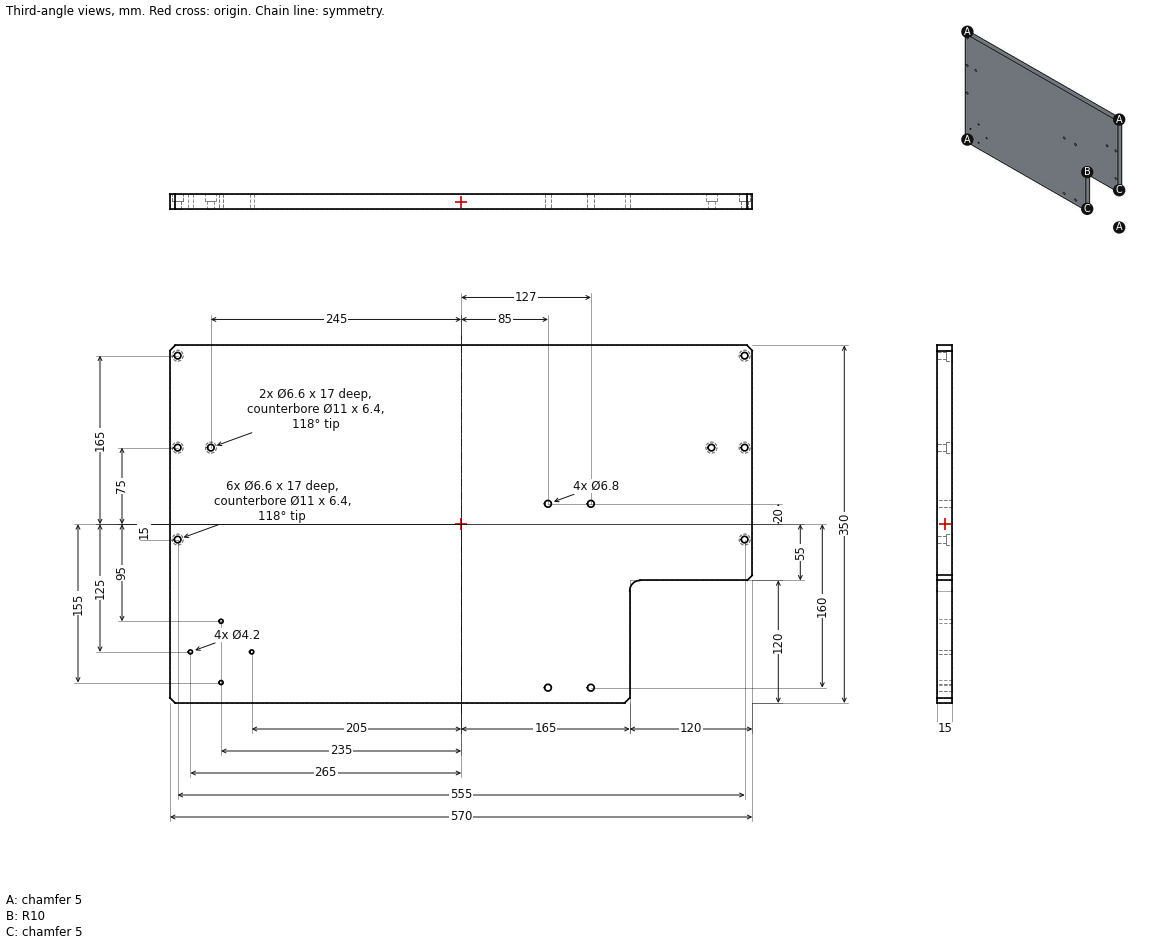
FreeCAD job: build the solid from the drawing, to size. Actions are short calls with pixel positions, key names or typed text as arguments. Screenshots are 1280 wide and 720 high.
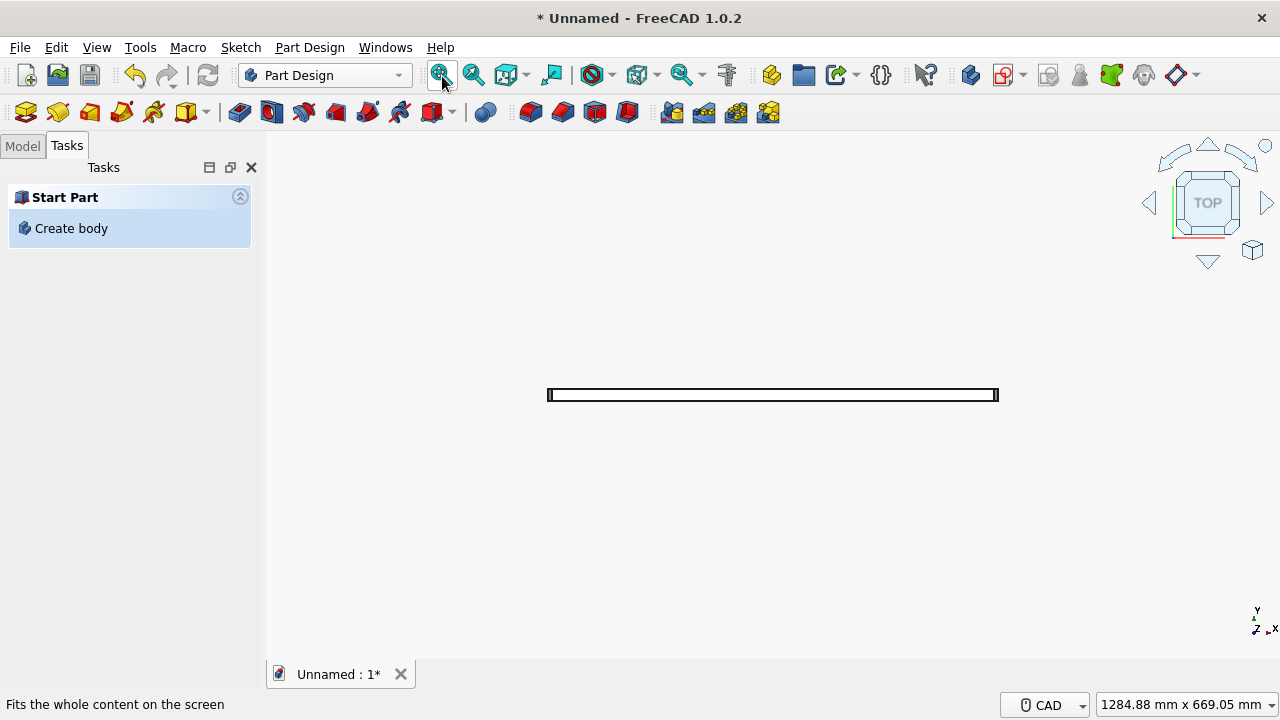
scroll(903, 394, up, 7)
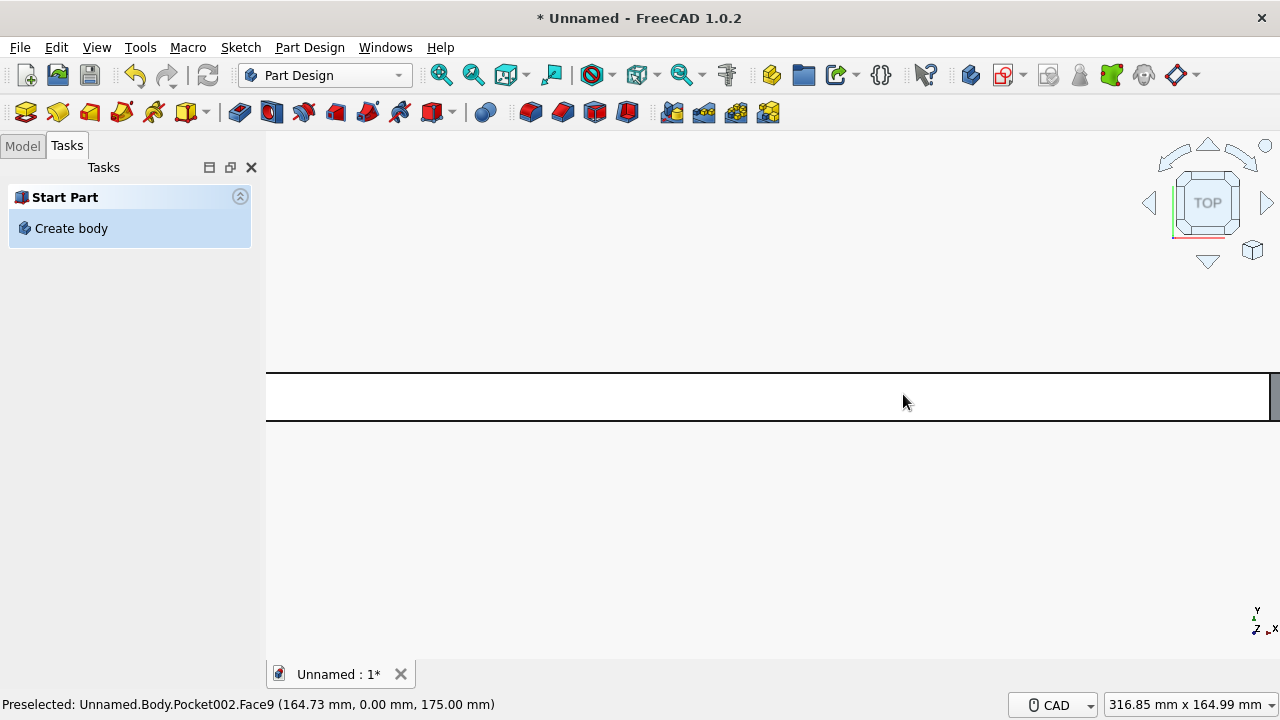
click(442, 76)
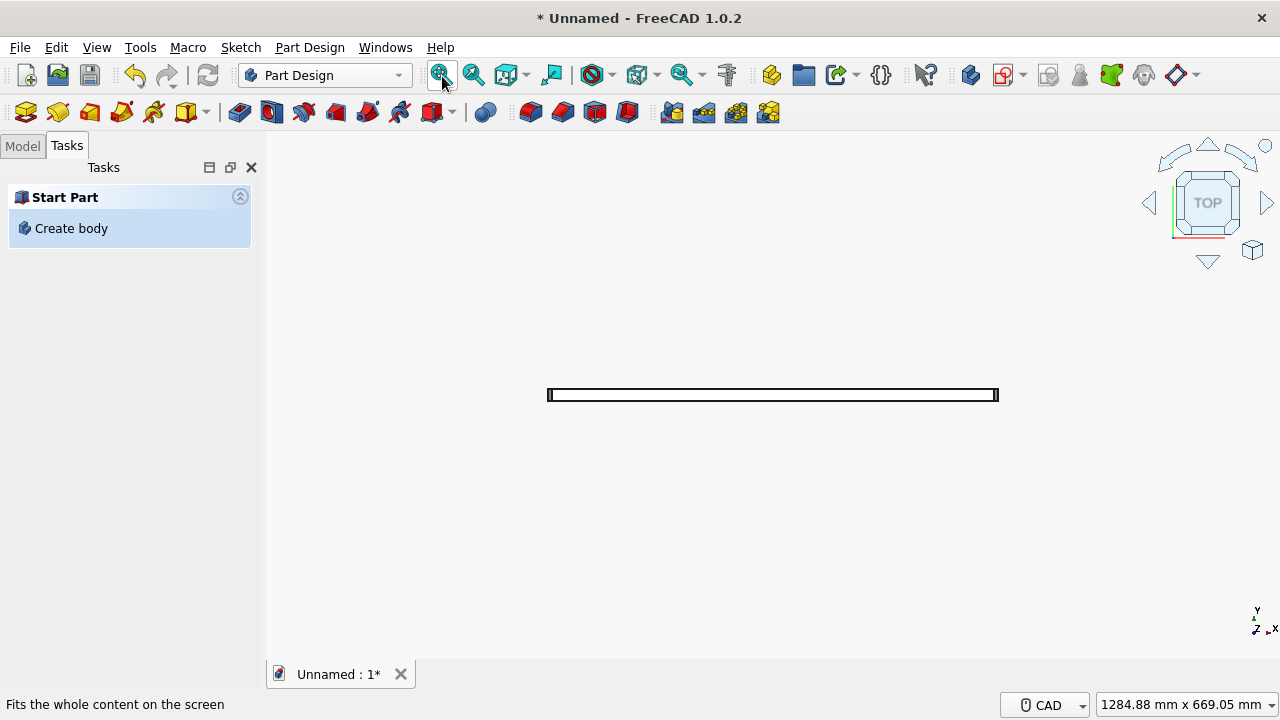
key(1)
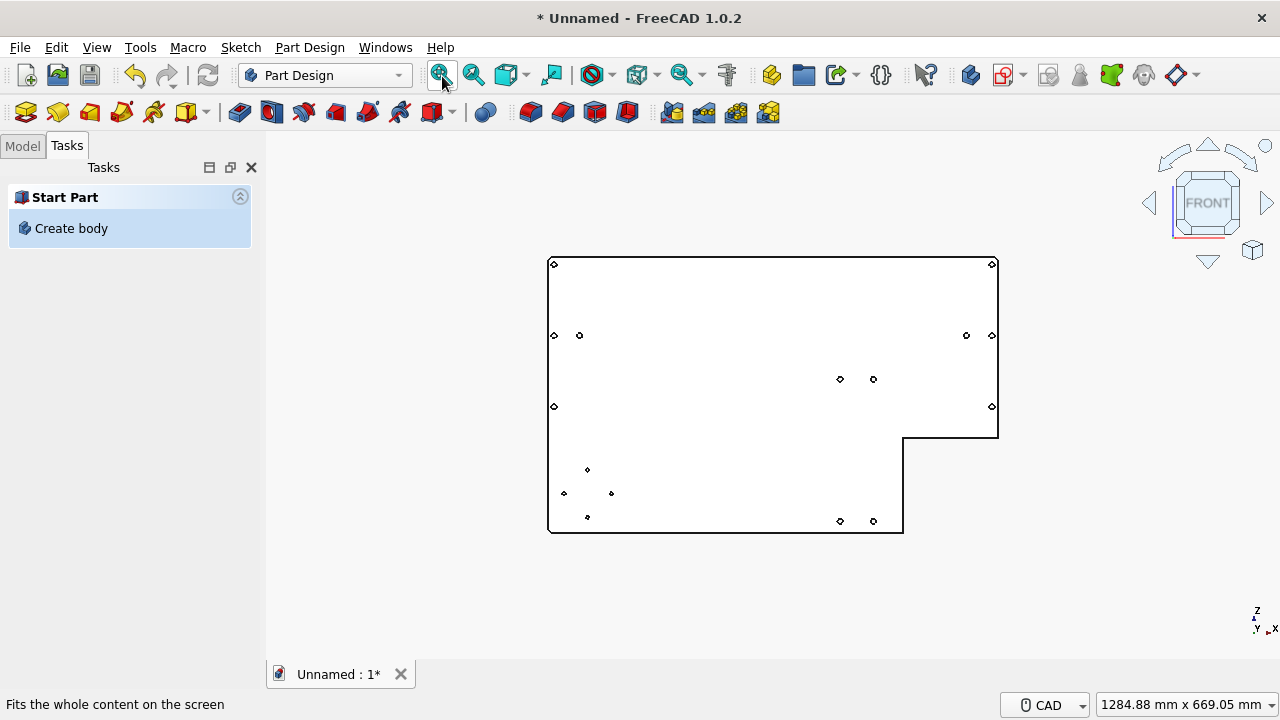
scroll(903, 437, up, 7)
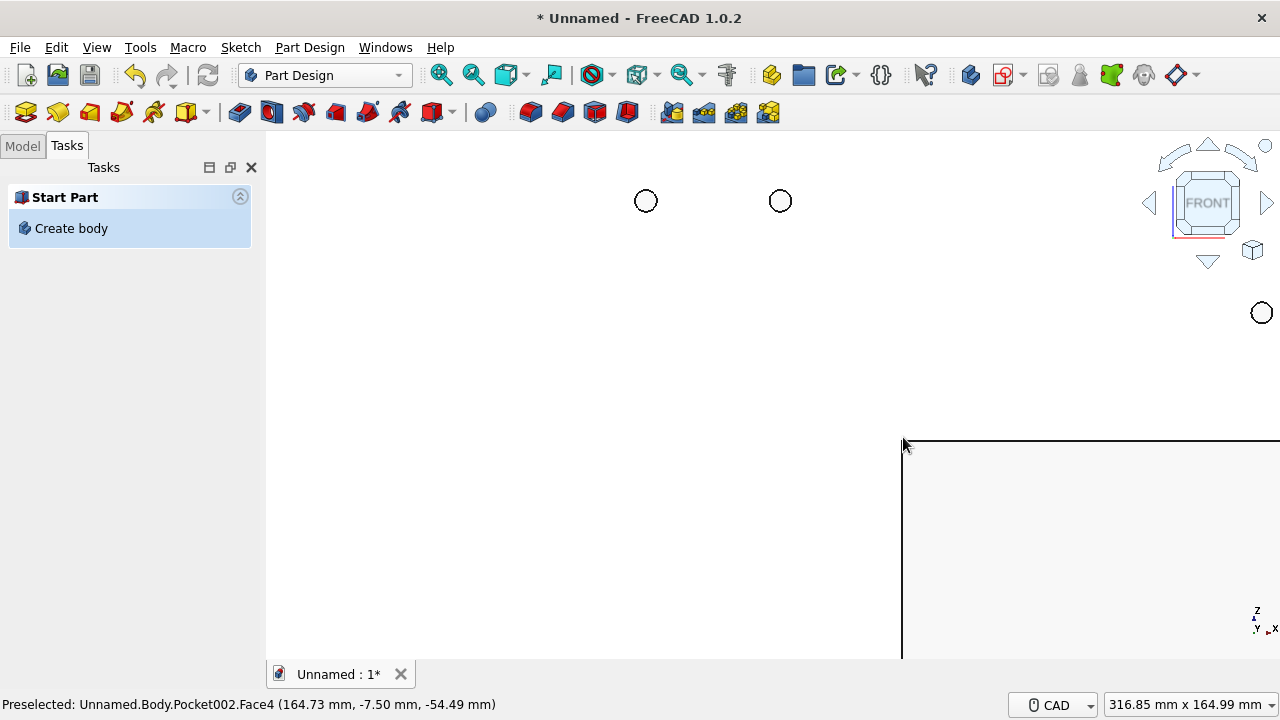
click(442, 76)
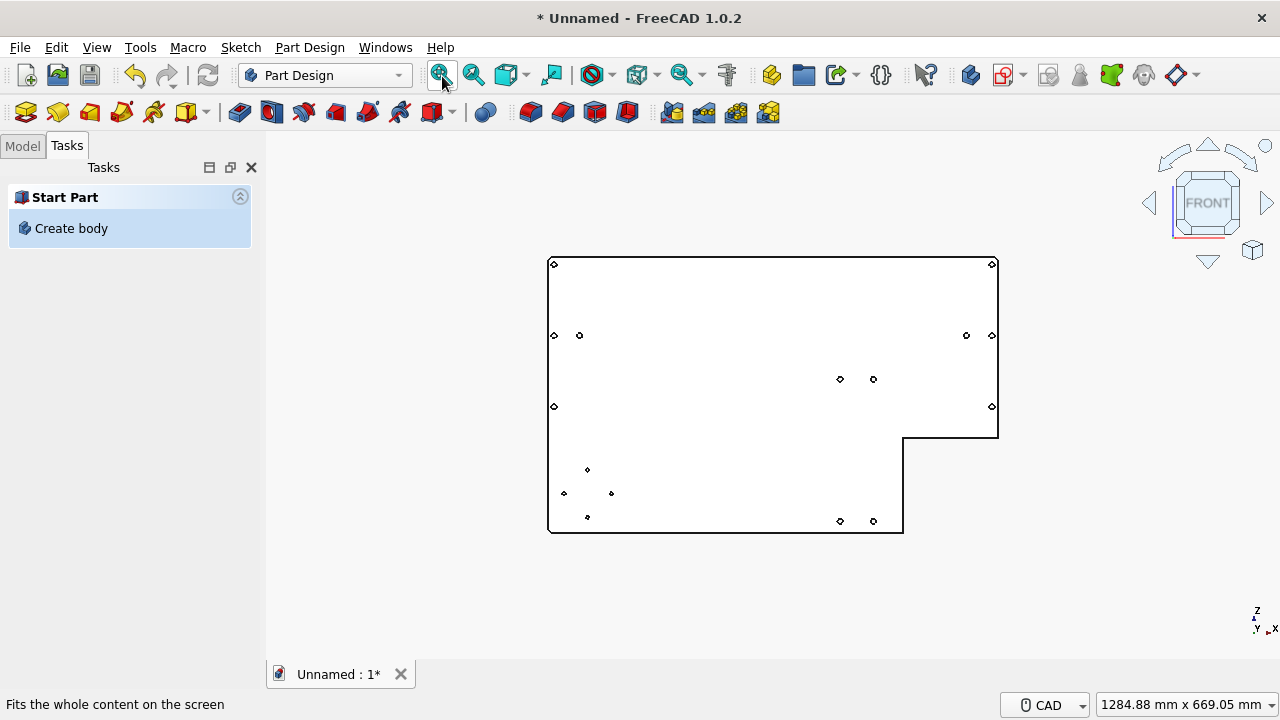
key(3)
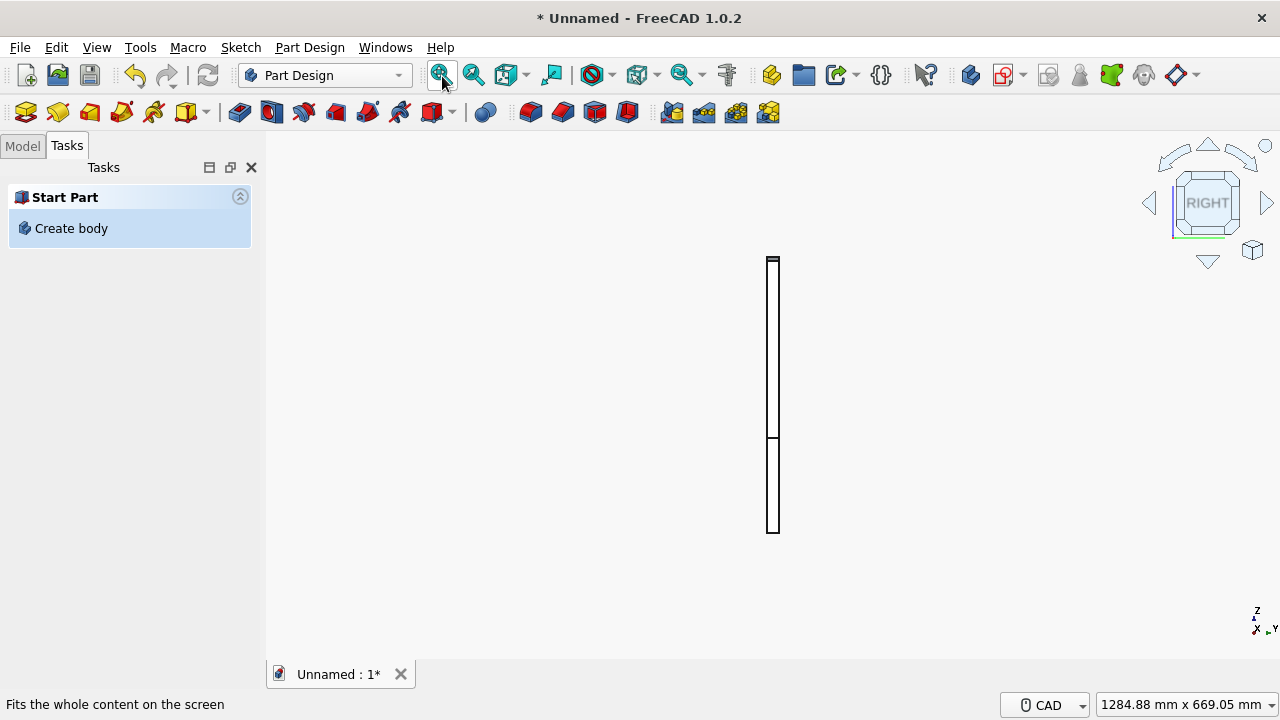
scroll(773, 437, up, 7)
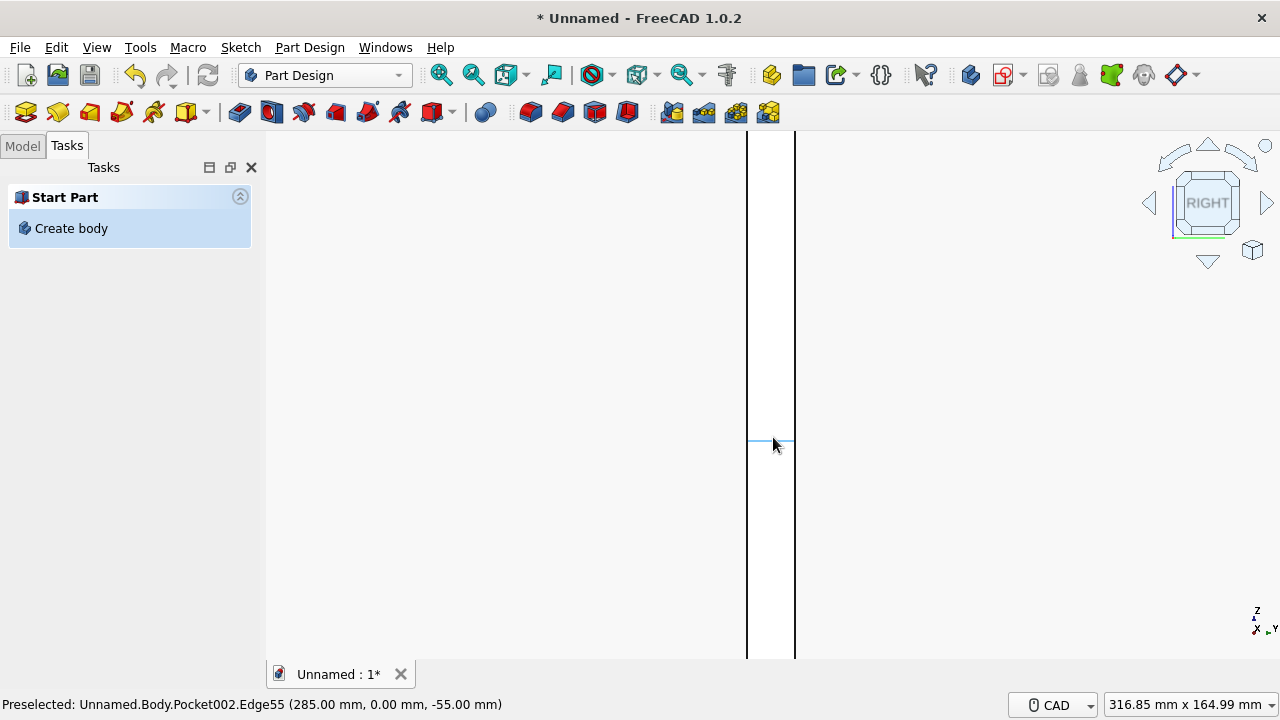
click(442, 76)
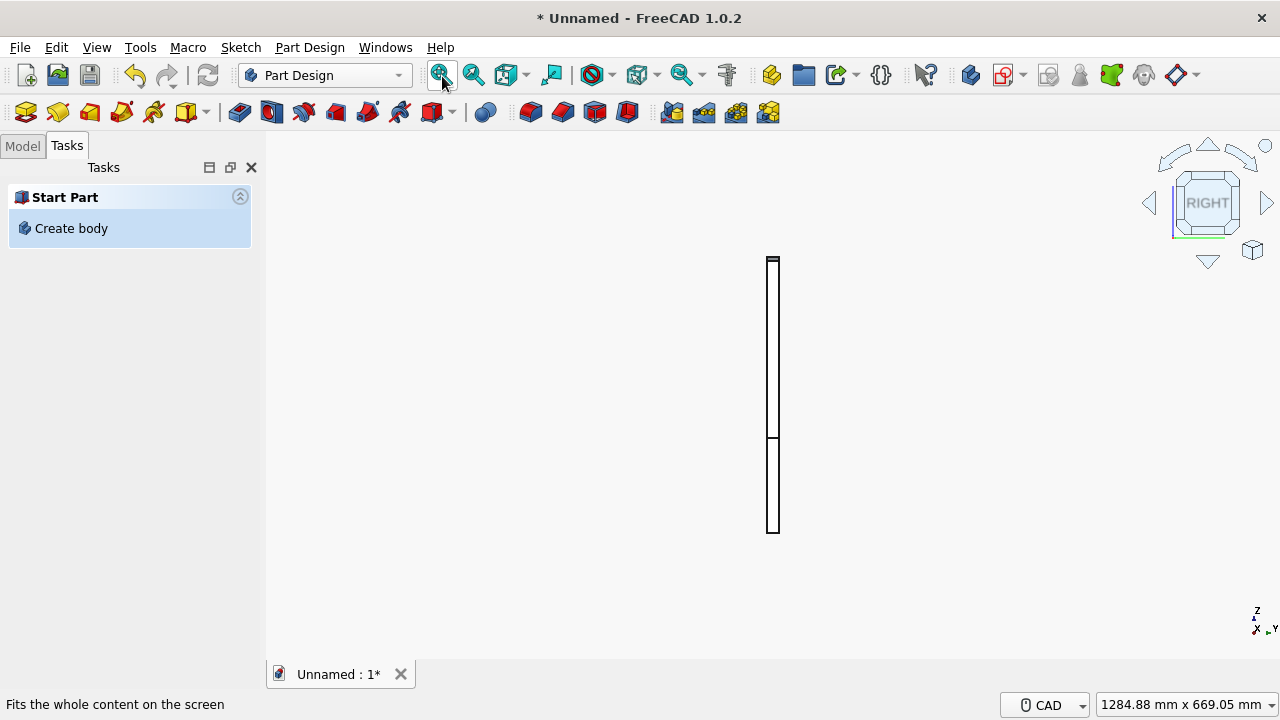
key(5)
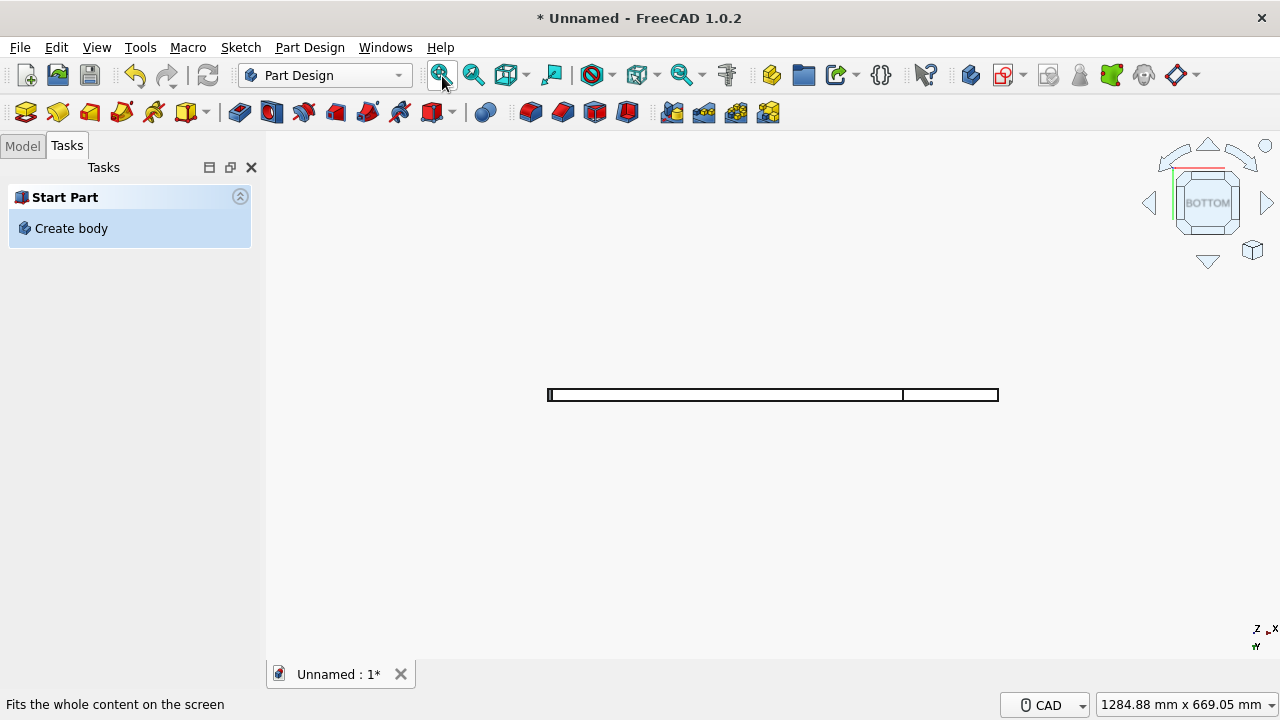
click(442, 76)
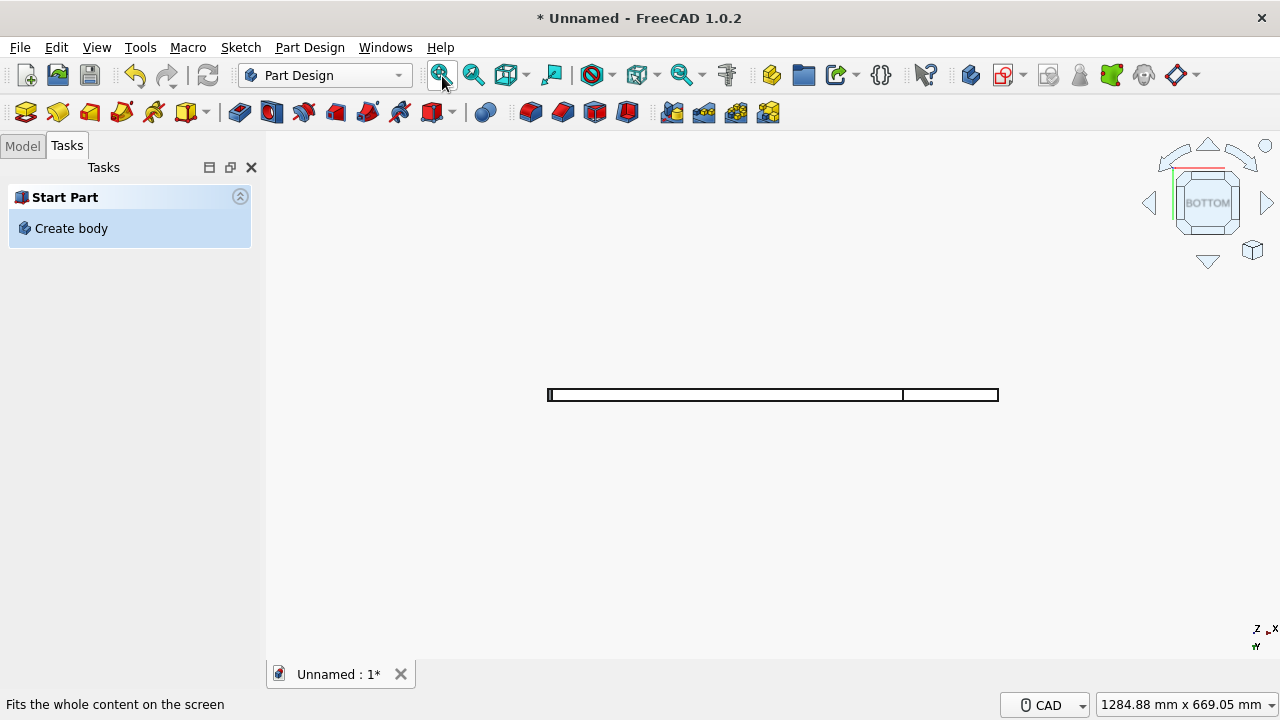
scroll(903, 394, up, 7)